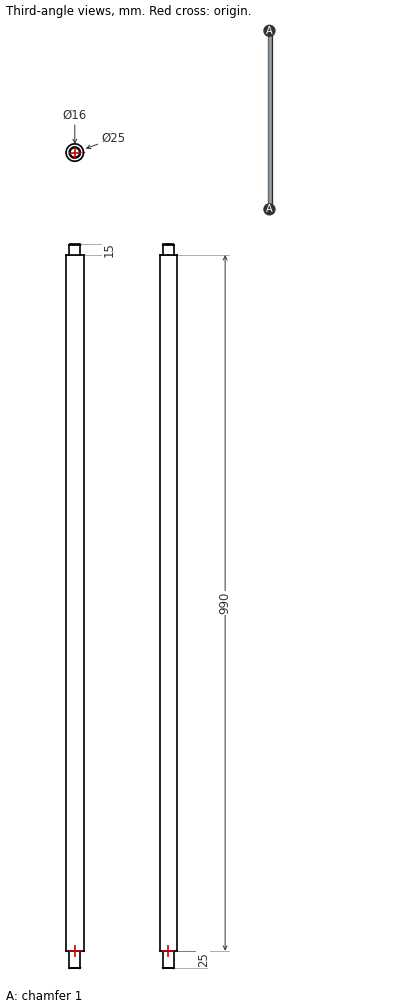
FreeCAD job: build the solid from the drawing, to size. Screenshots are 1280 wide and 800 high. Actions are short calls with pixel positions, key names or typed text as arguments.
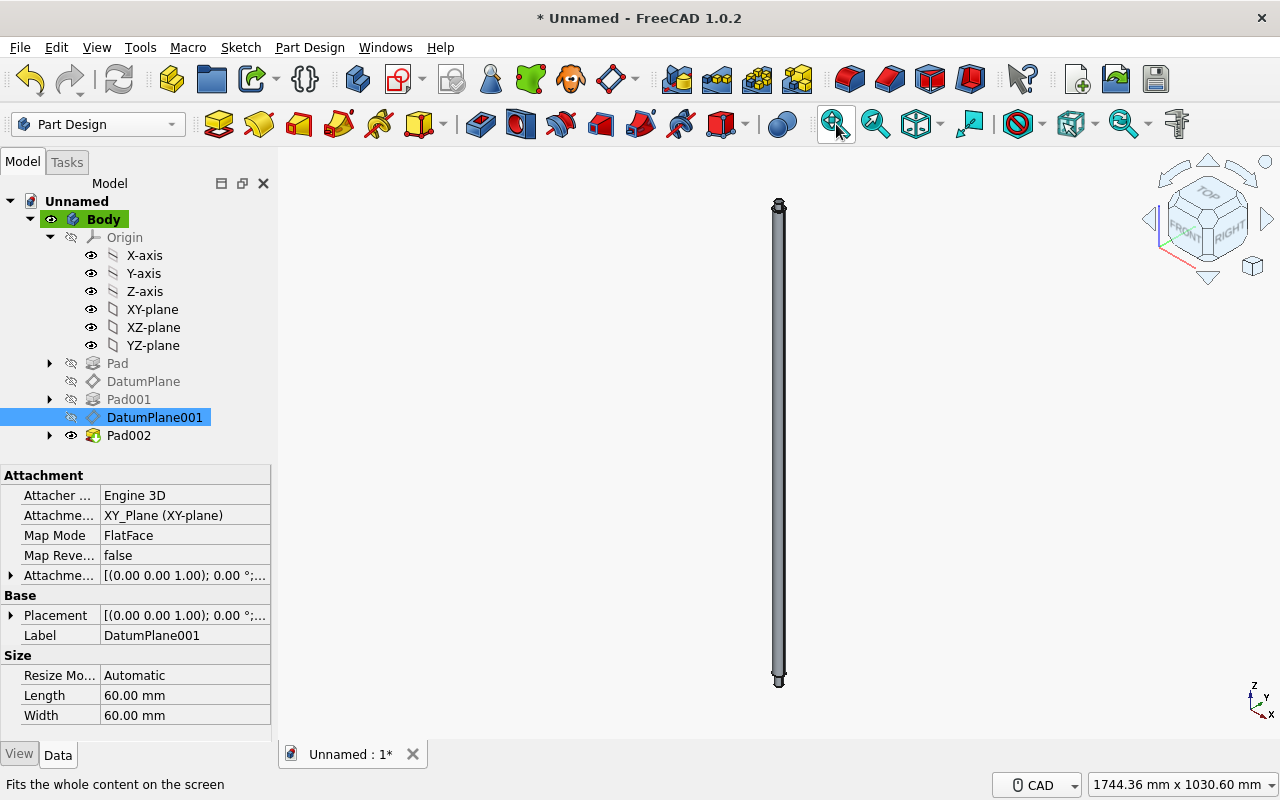
click(776, 199)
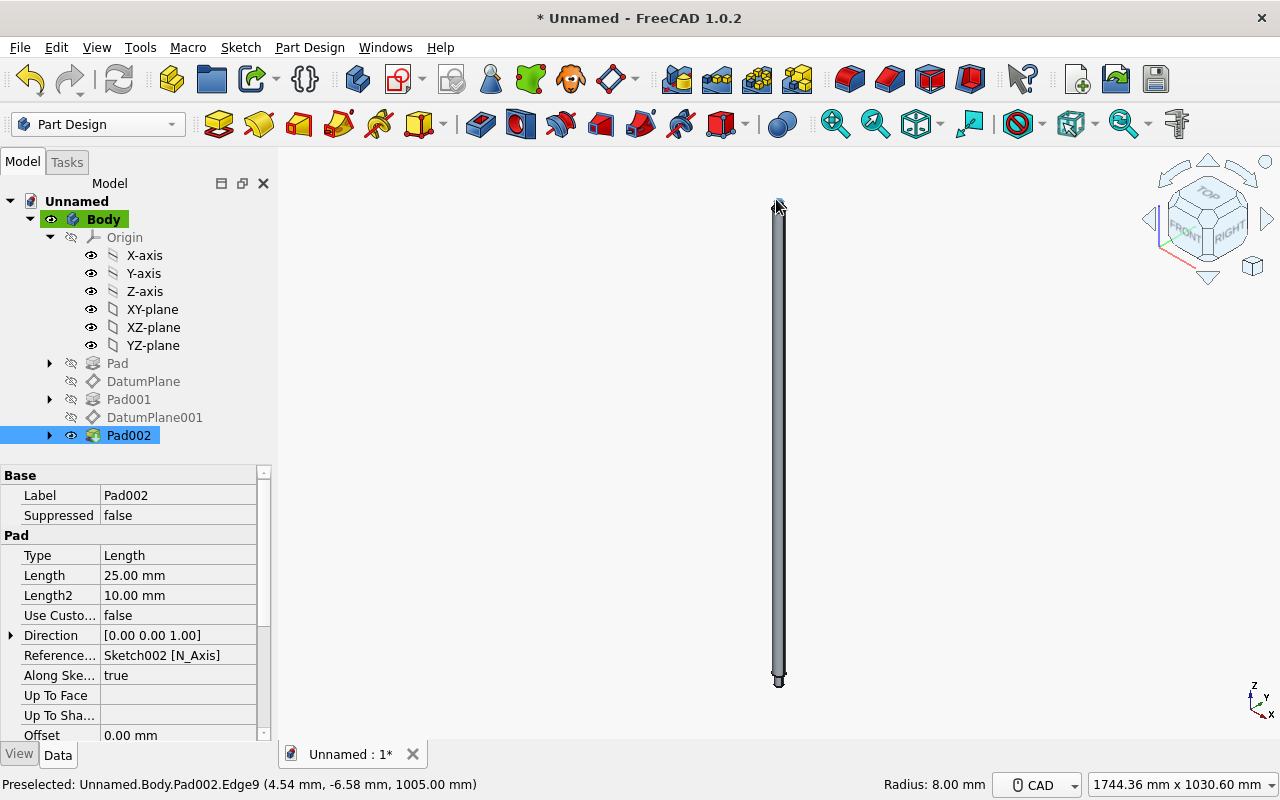
key(2)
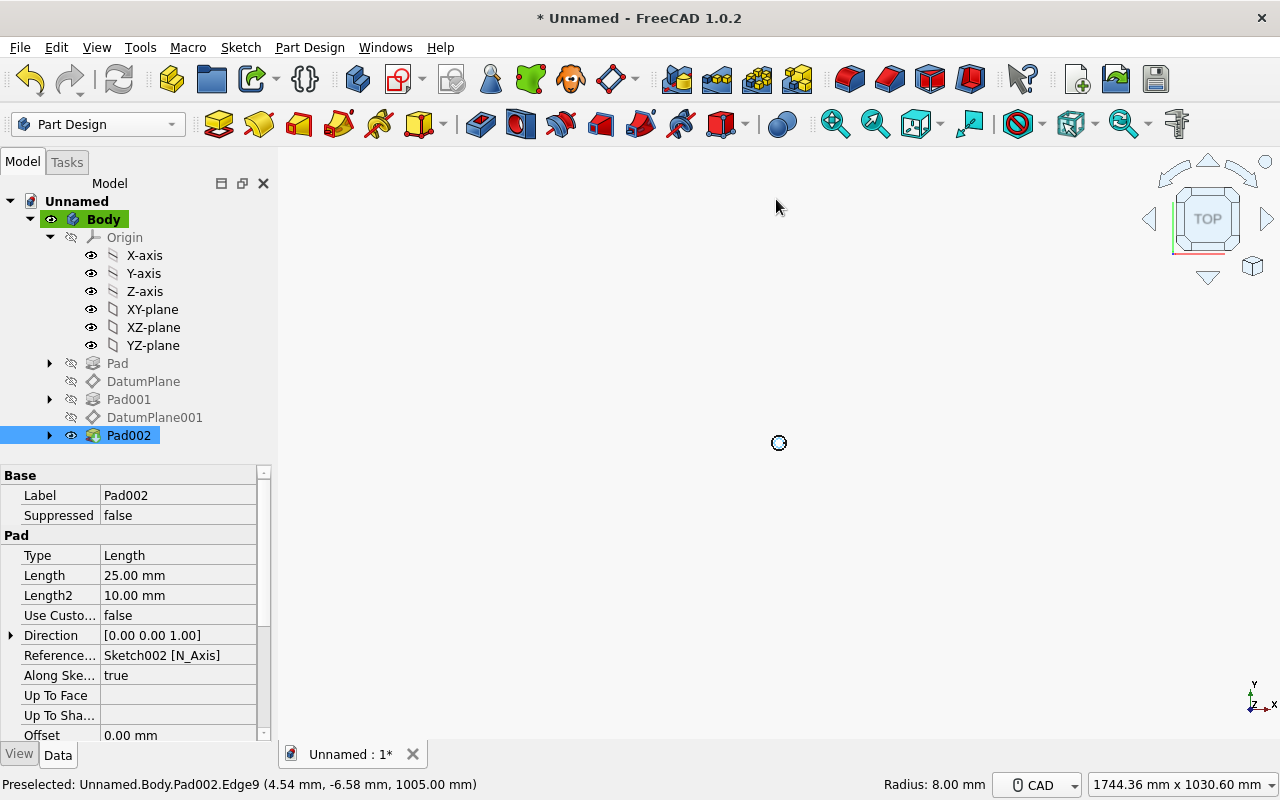
click(836, 124)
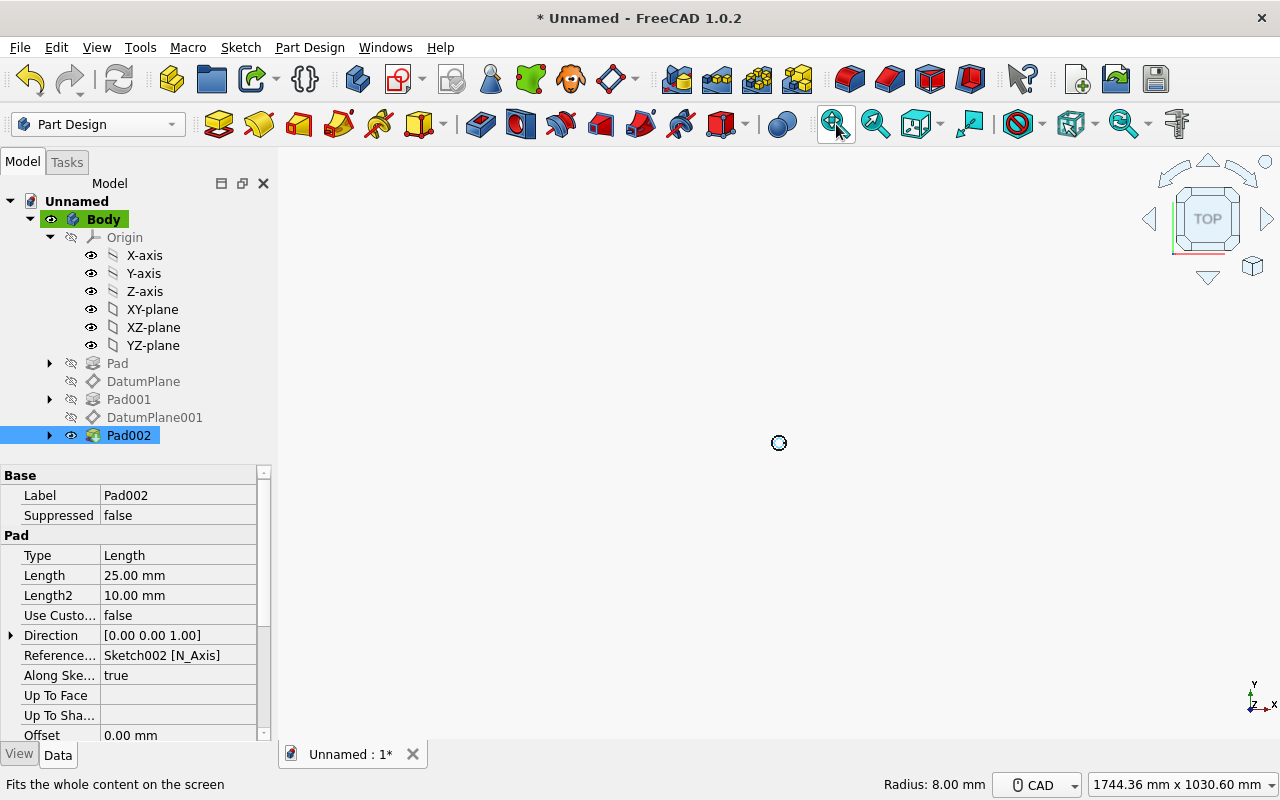
key(1)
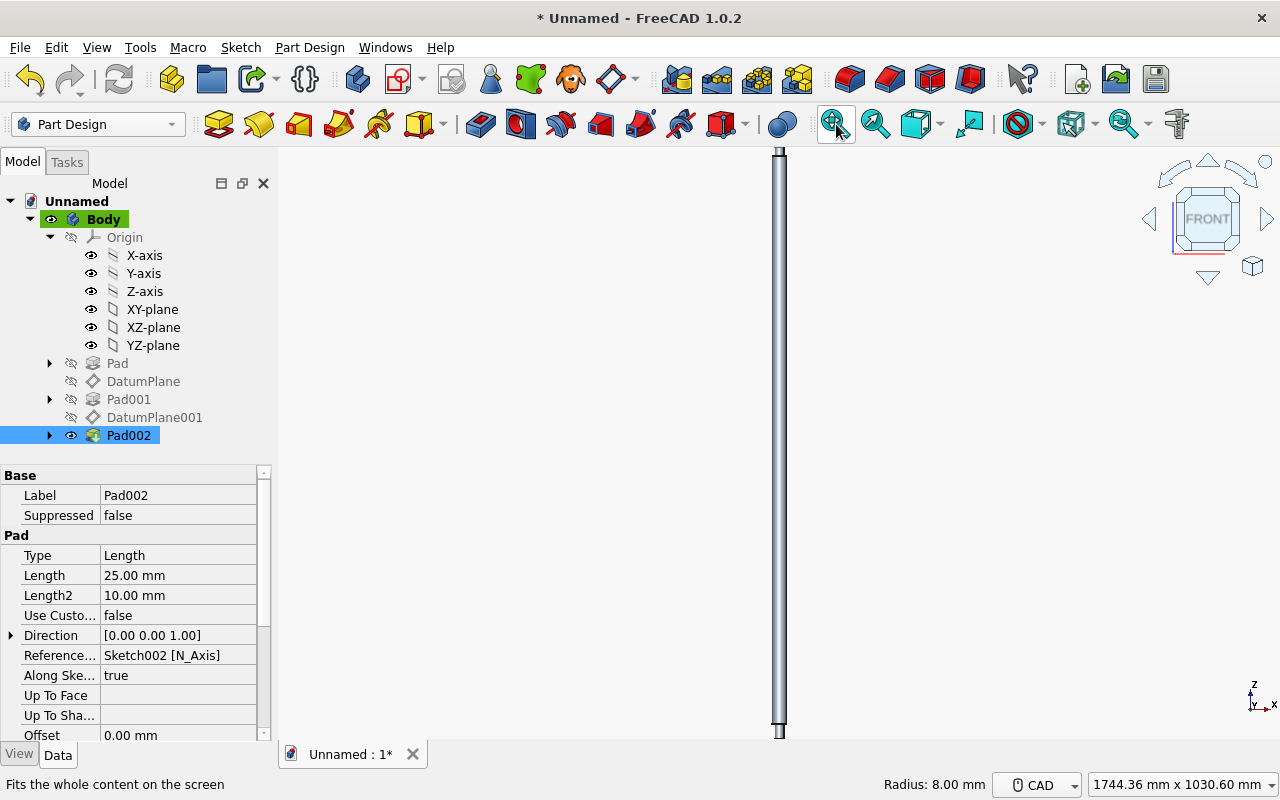
click(836, 124)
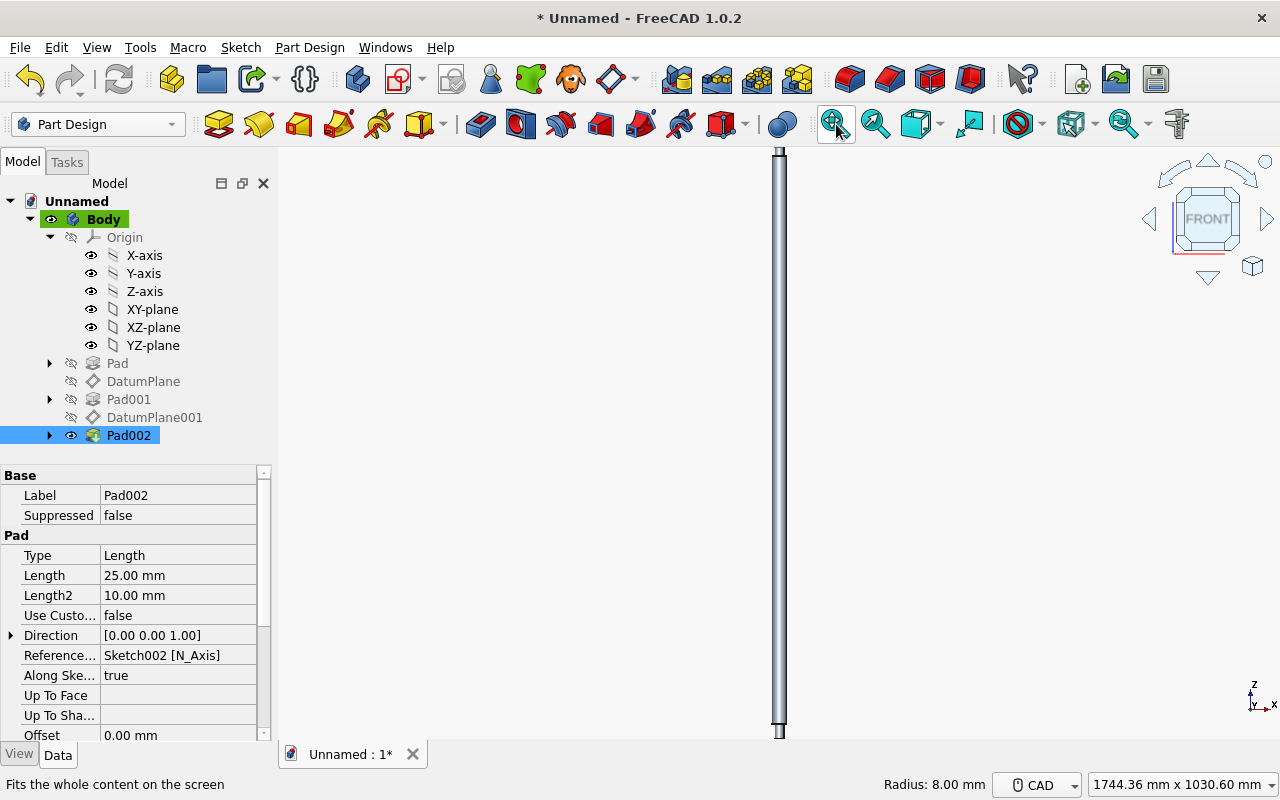
key(3)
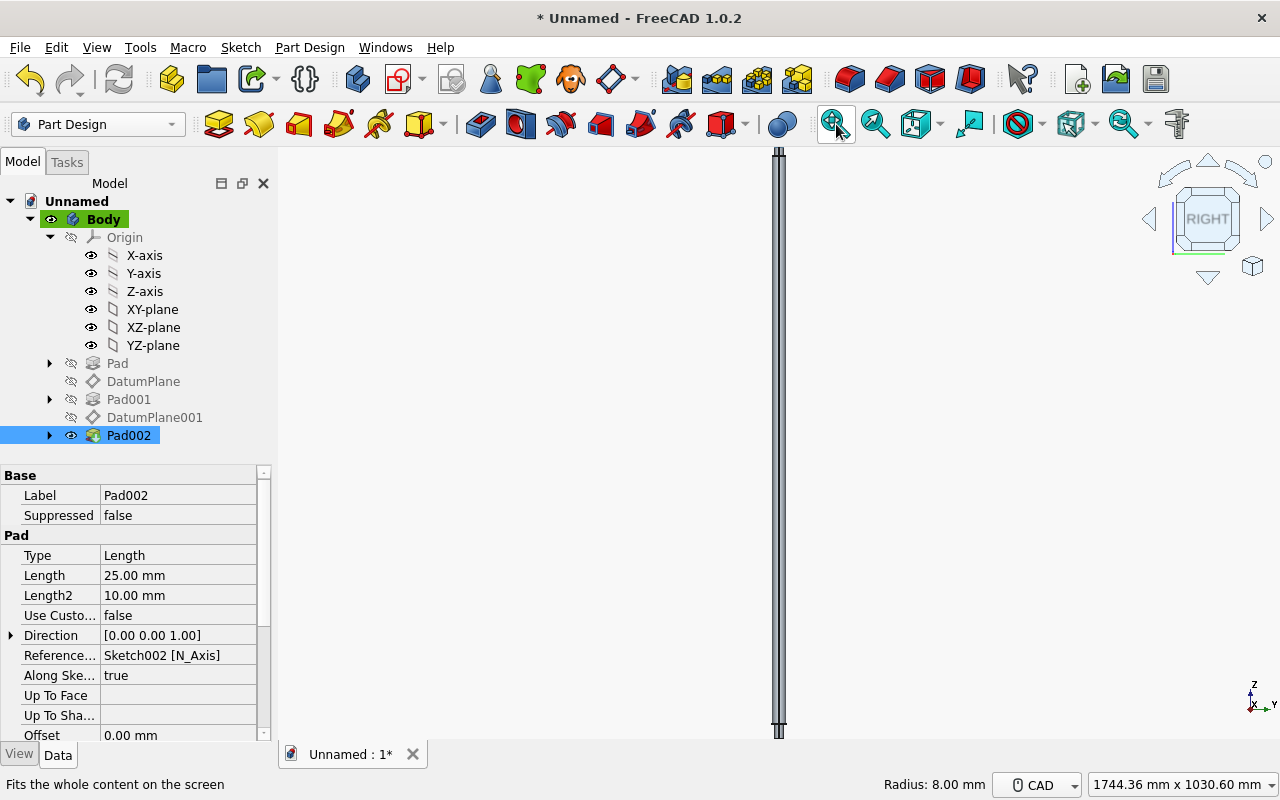
click(836, 124)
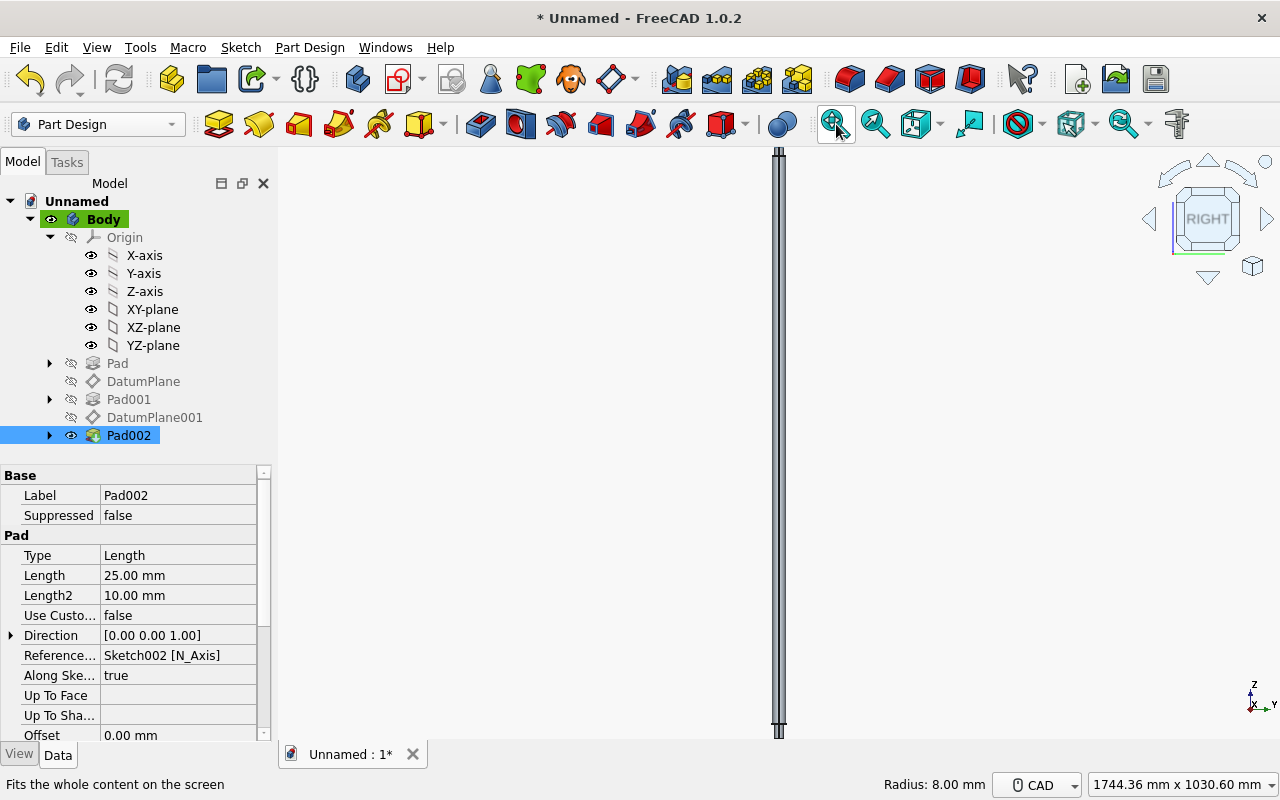
key(5)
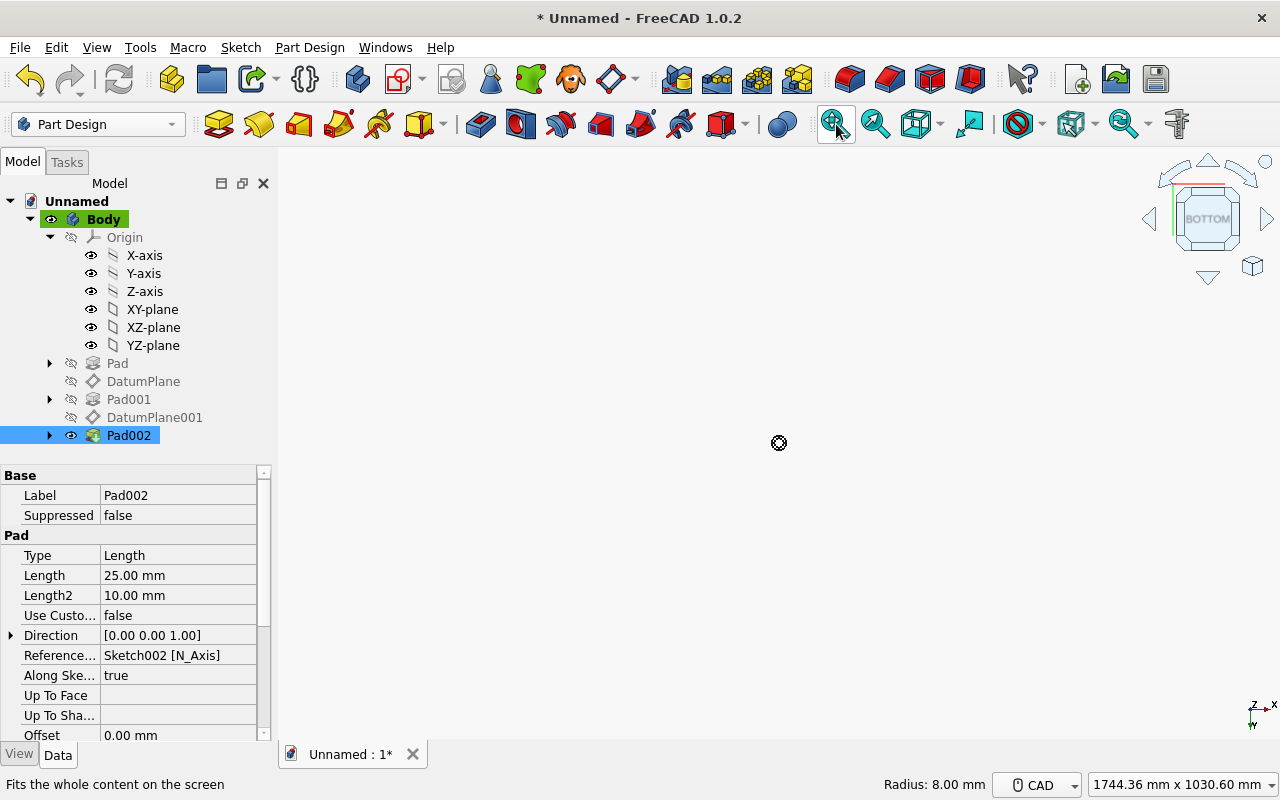
click(836, 124)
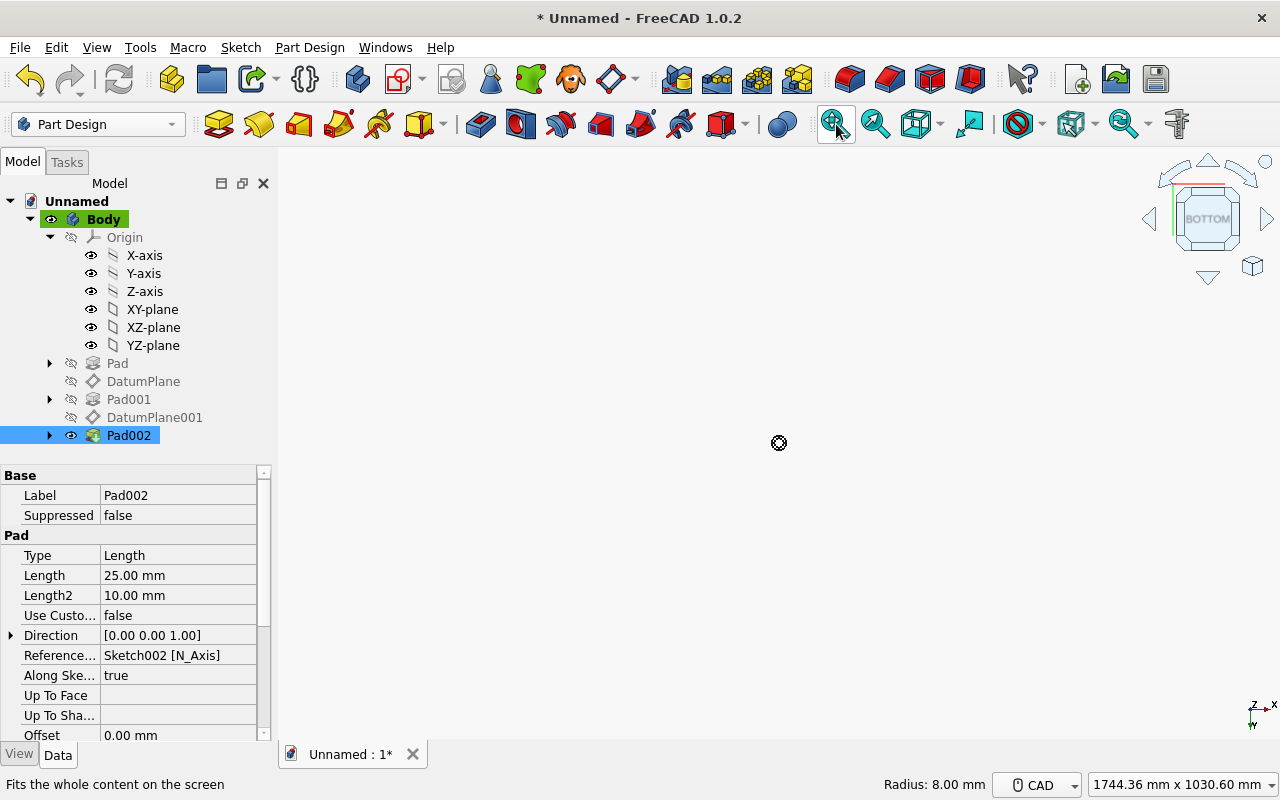
click(774, 442, ctrl)